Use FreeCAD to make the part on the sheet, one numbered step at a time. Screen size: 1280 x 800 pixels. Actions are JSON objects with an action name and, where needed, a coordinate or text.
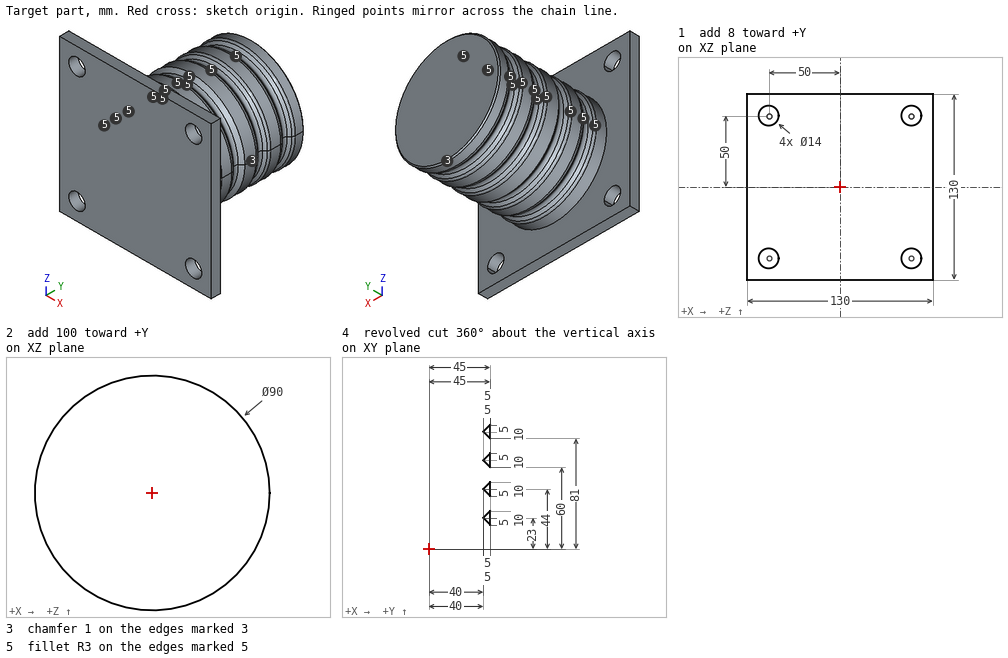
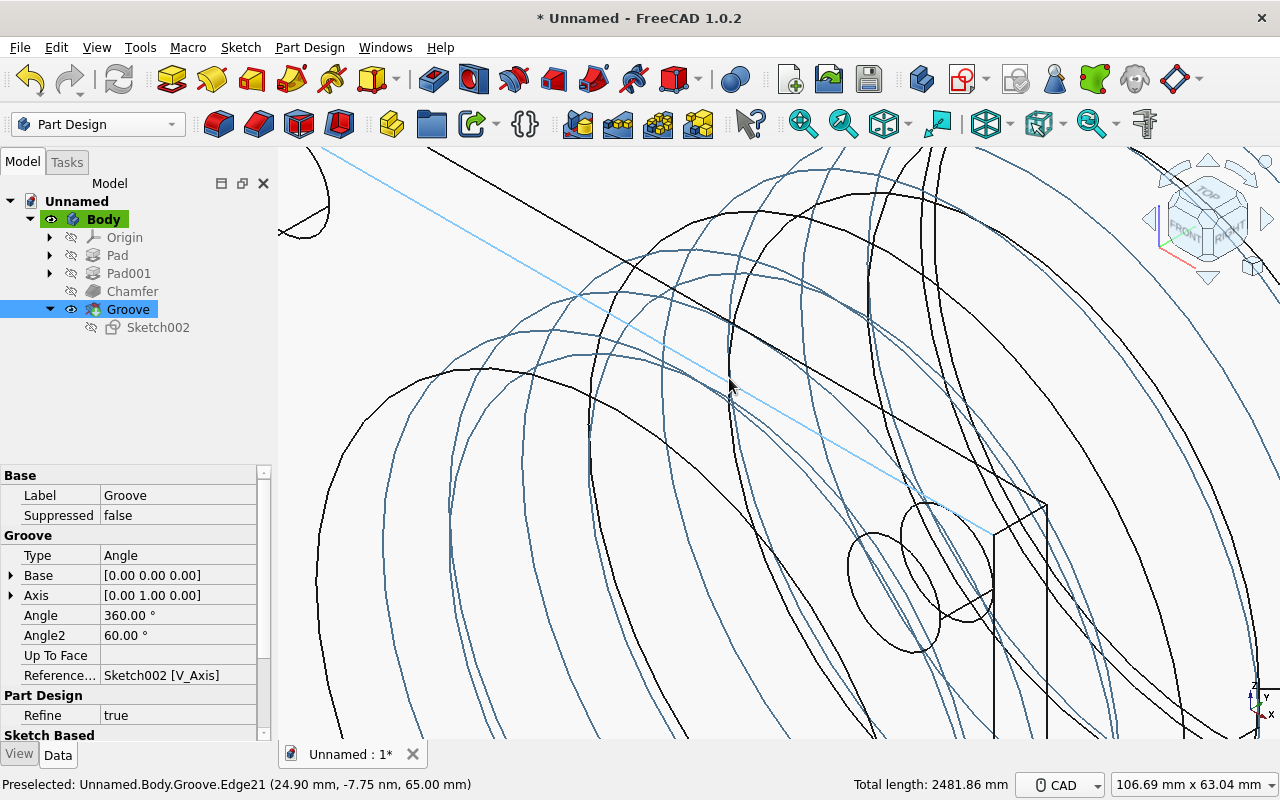
{"action": "left_click", "coordinate": [779, 591], "text": "ctrl"}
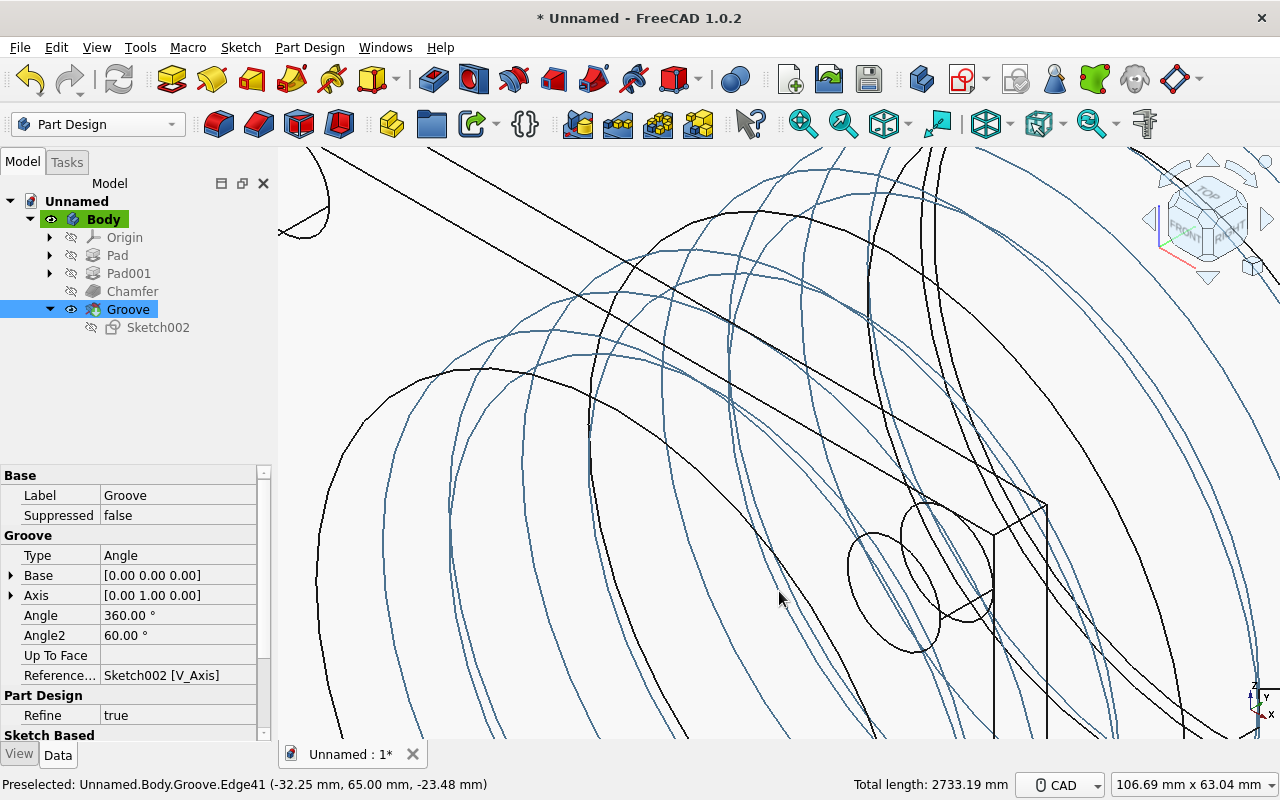
{"action": "left_click", "coordinate": [867, 301], "text": "ctrl"}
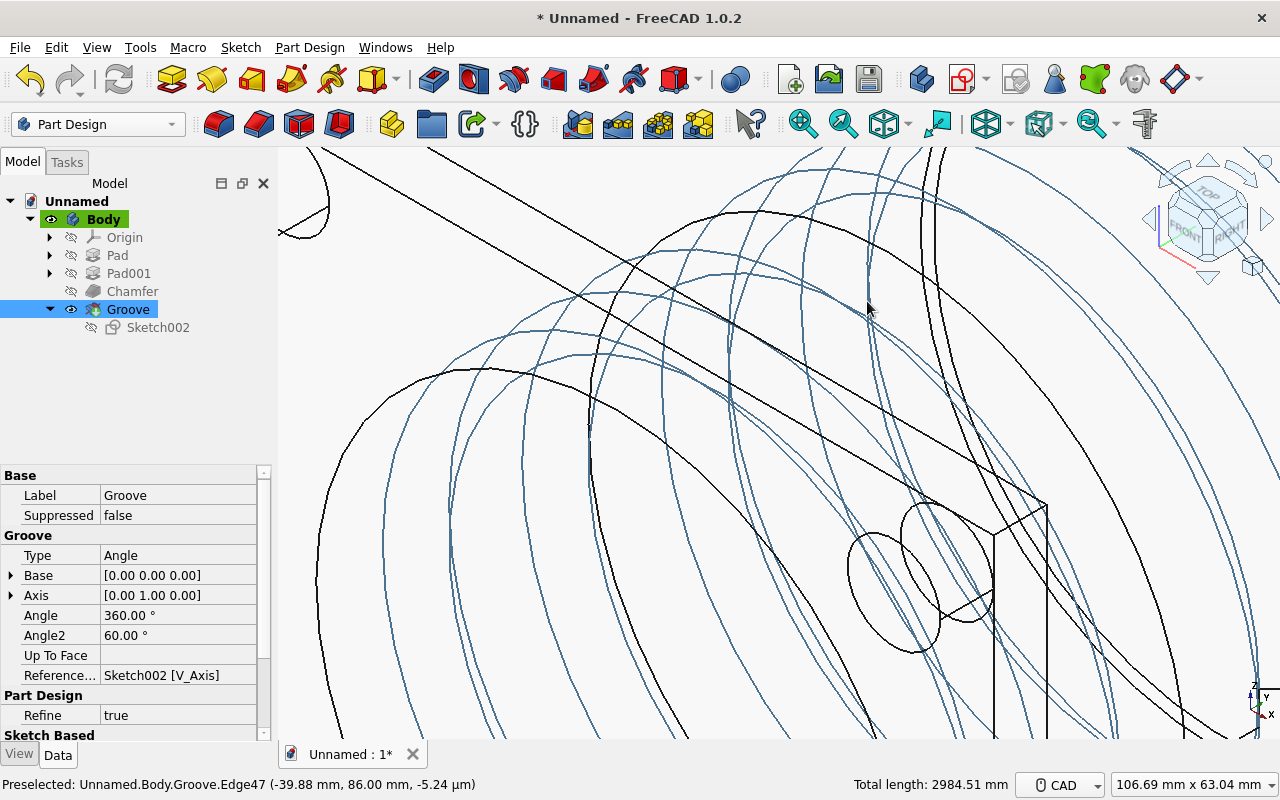
{"action": "key", "text": "v 1"}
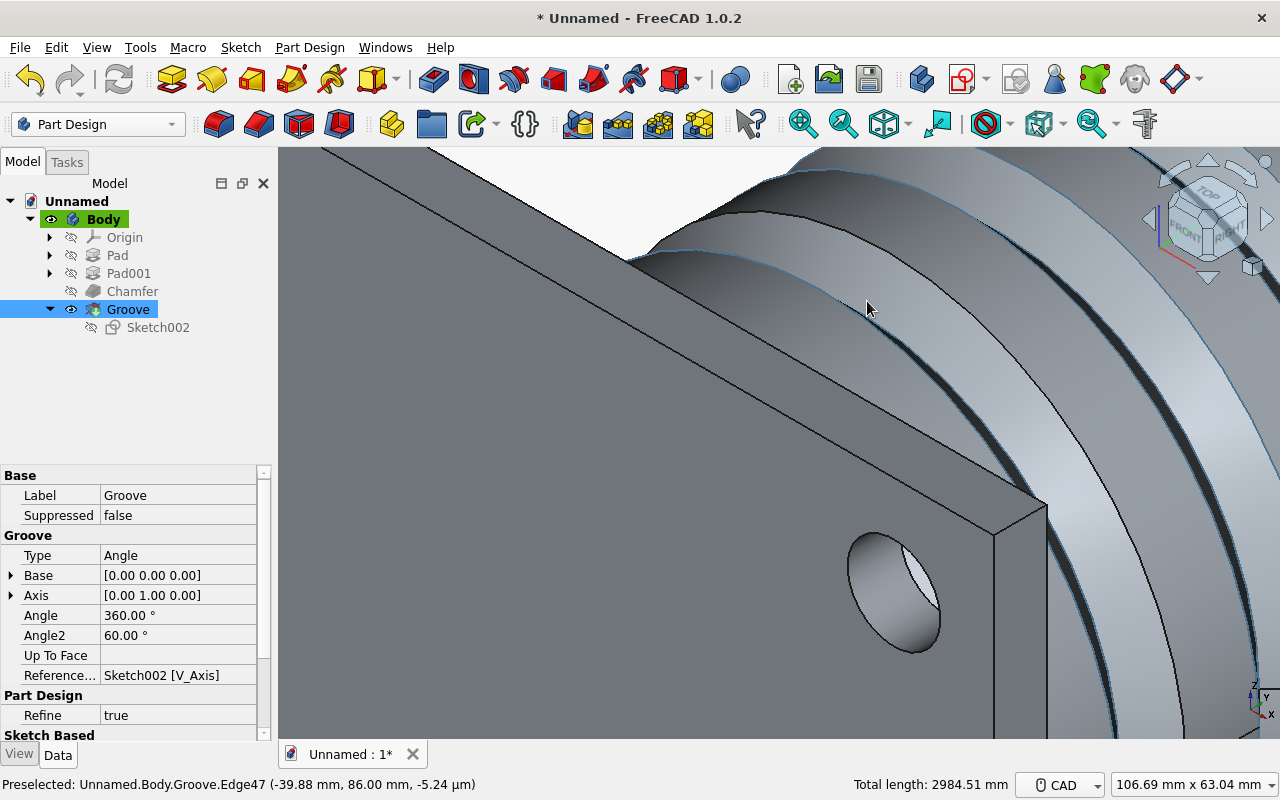
{"action": "left_click", "coordinate": [220, 124]}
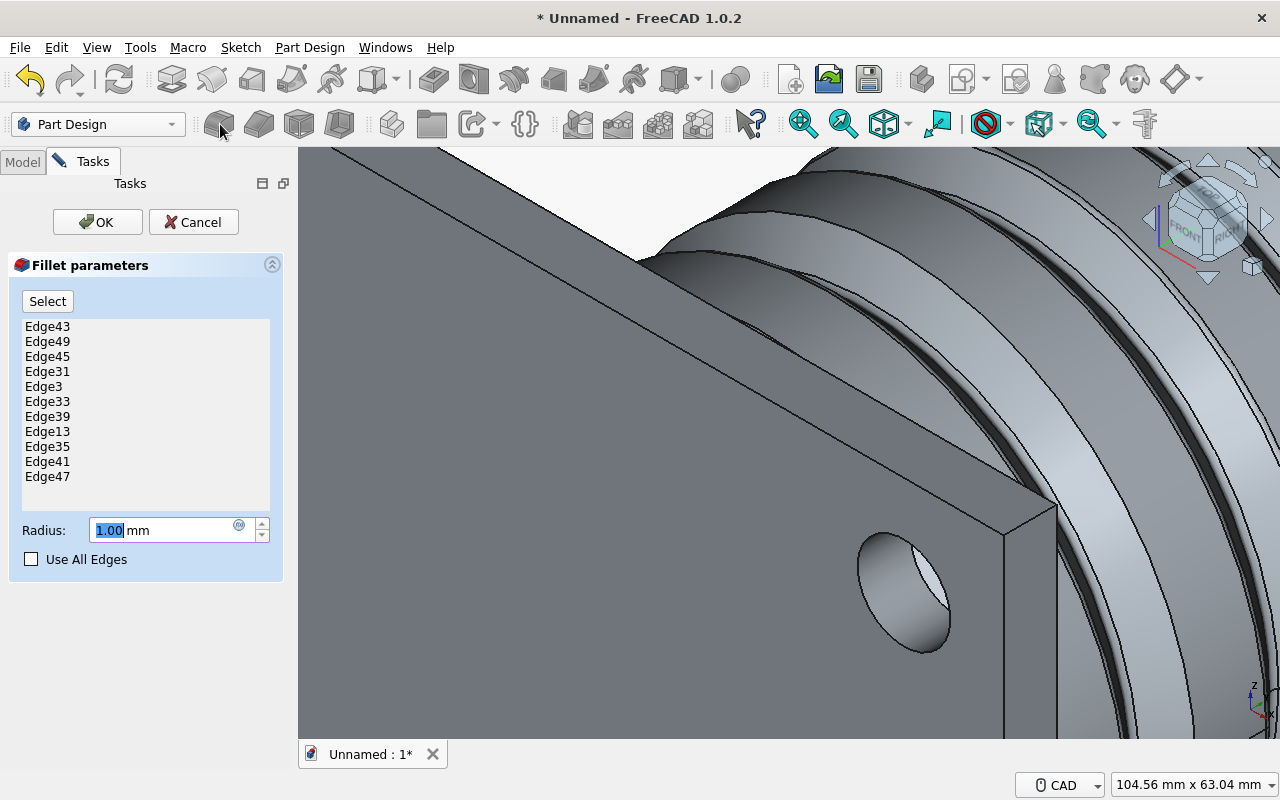
{"action": "type", "text": "3"}
{"action": "key", "text": "Tab"}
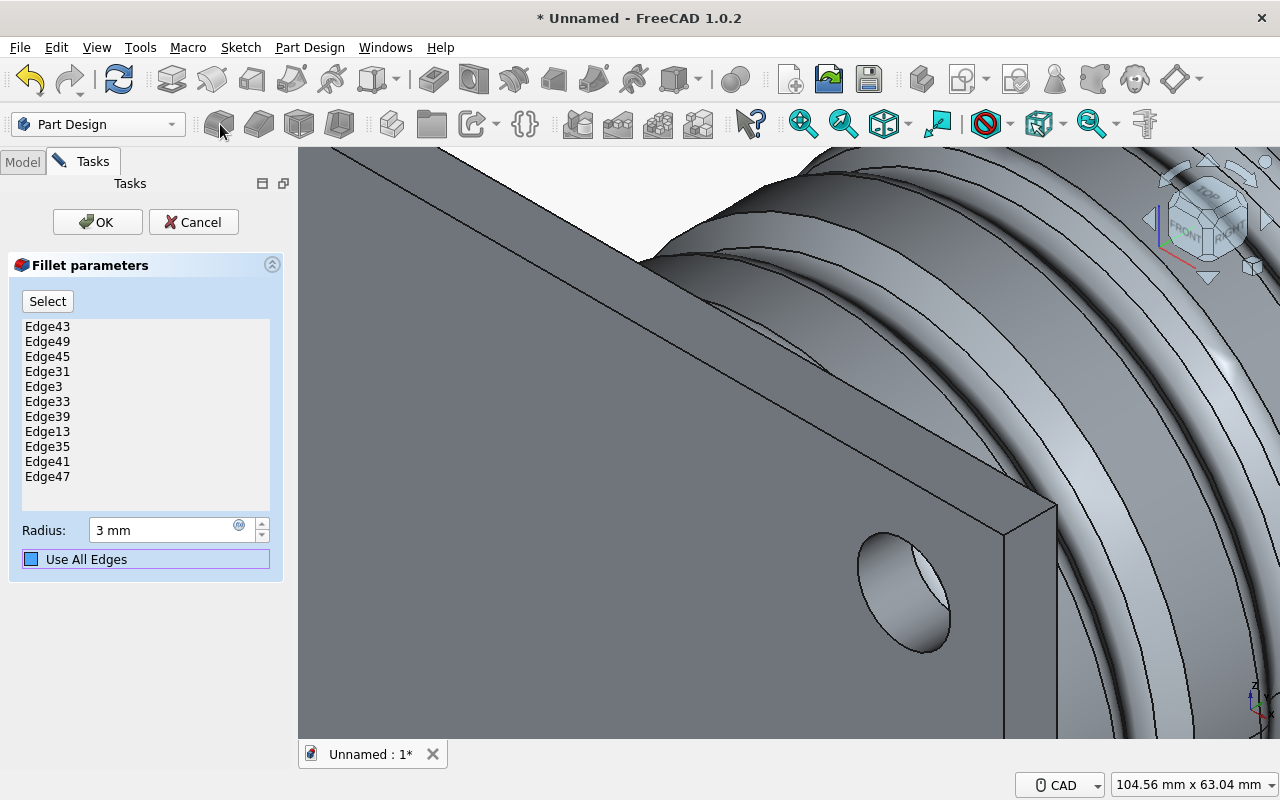
{"action": "left_click", "coordinate": [98, 222]}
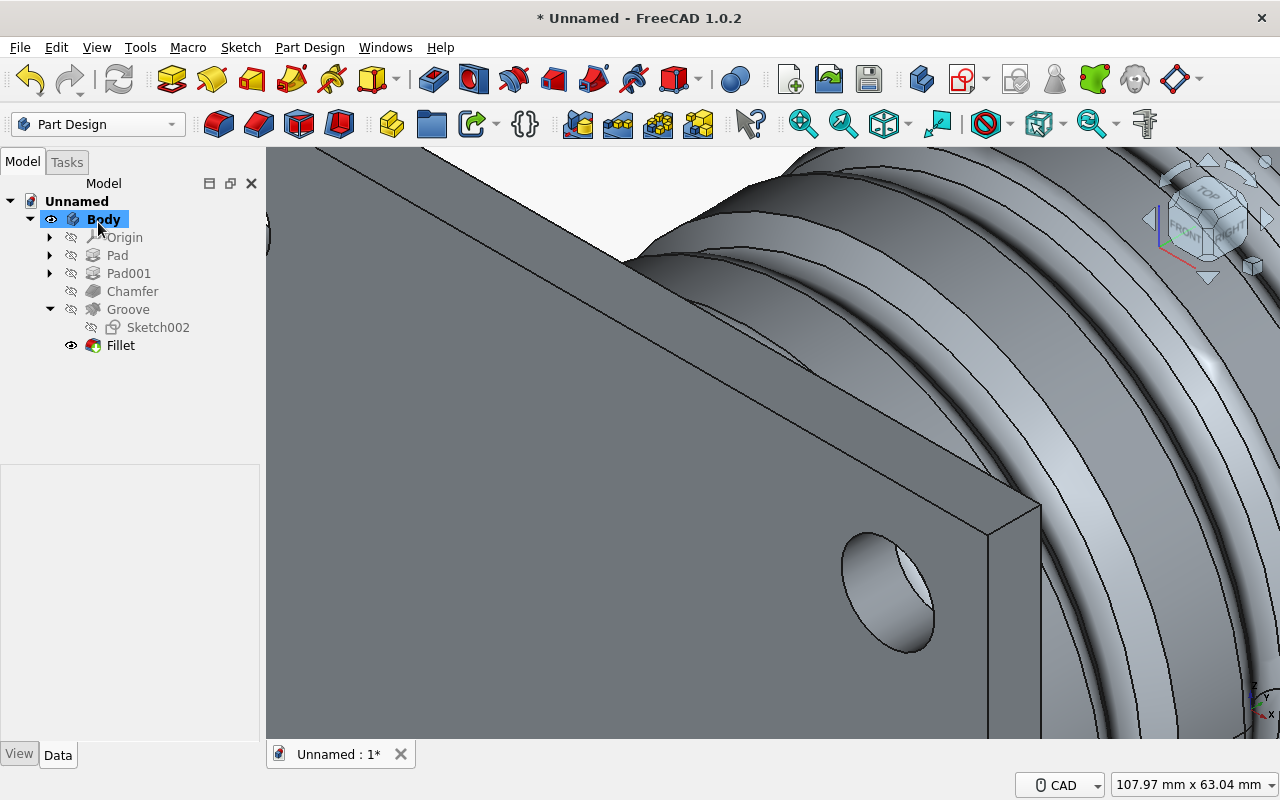
{"action": "left_click", "coordinate": [804, 124]}